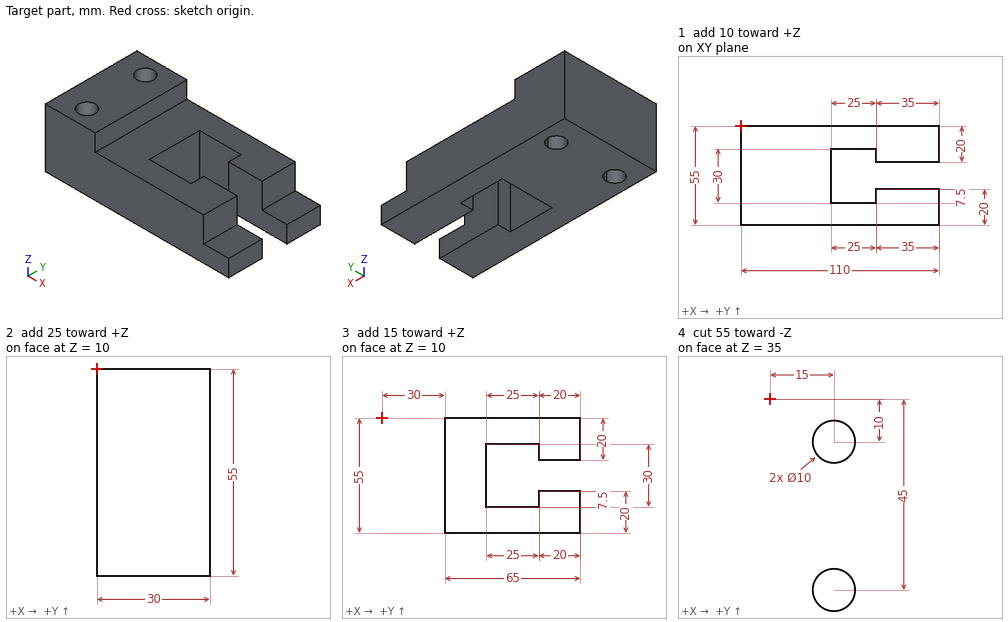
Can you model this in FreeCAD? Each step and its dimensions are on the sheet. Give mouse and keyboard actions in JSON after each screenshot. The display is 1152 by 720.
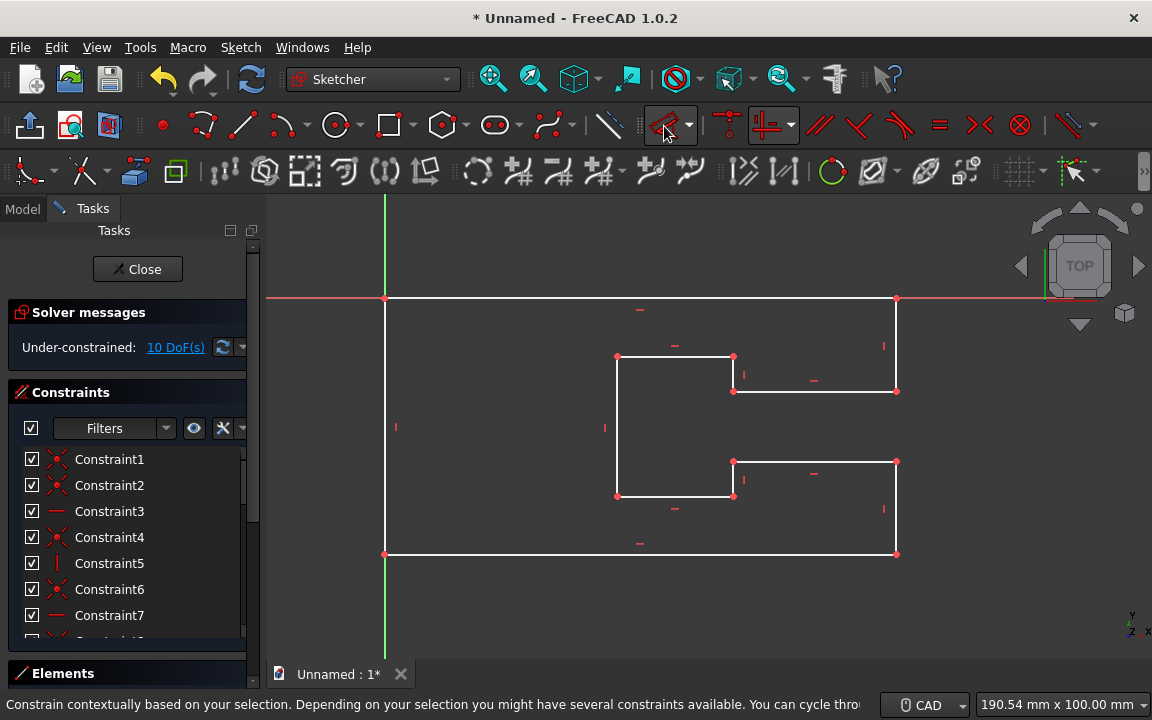
{"action": "left_click", "coordinate": [385, 375]}
{"action": "left_click", "coordinate": [351, 427]}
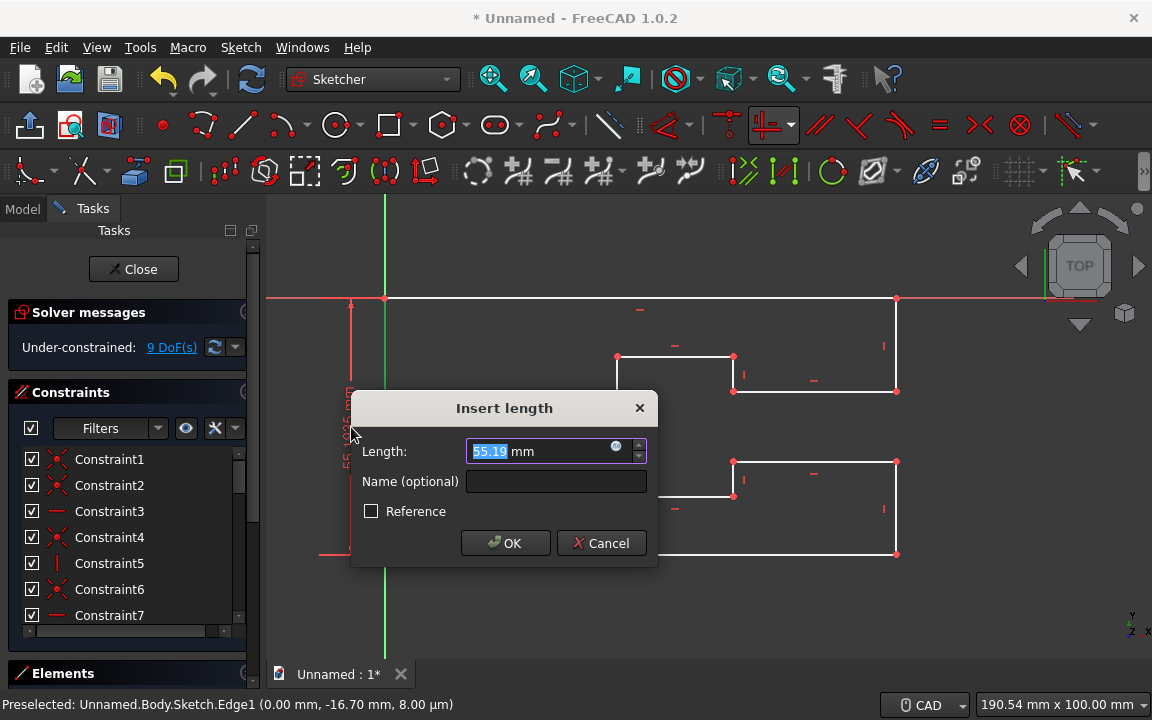
{"action": "type", "text": "55"}
{"action": "key", "text": "Return"}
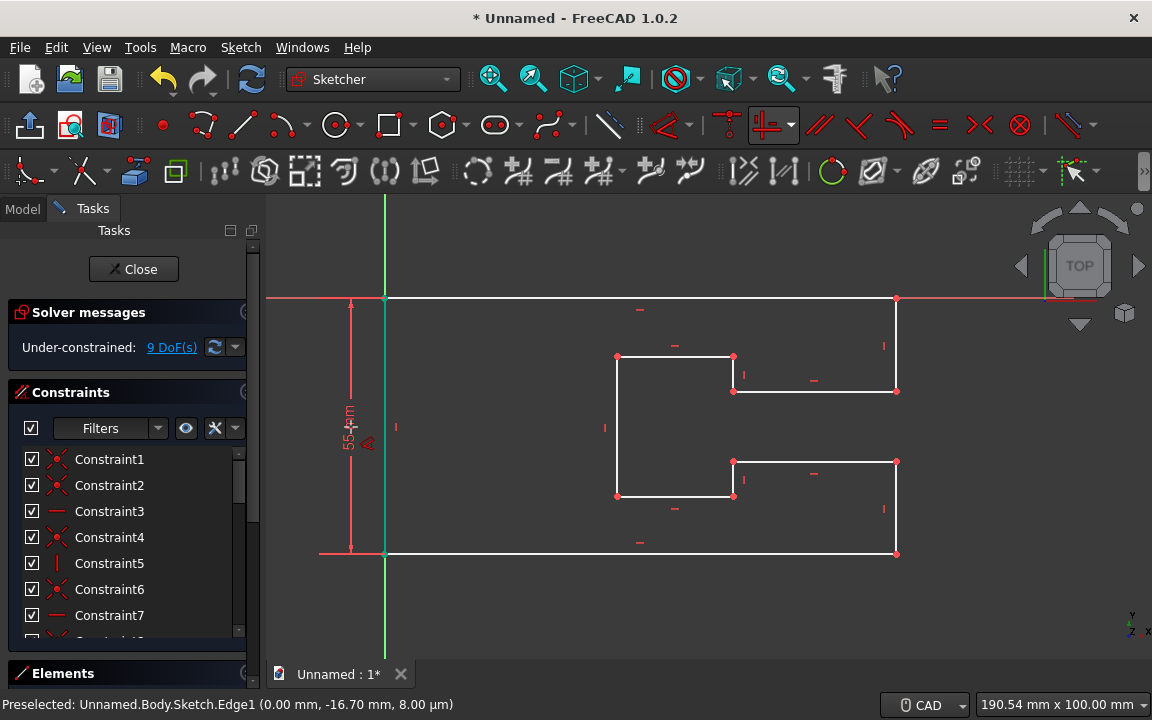
{"action": "left_click", "coordinate": [896, 526]}
{"action": "left_click", "coordinate": [930, 508]}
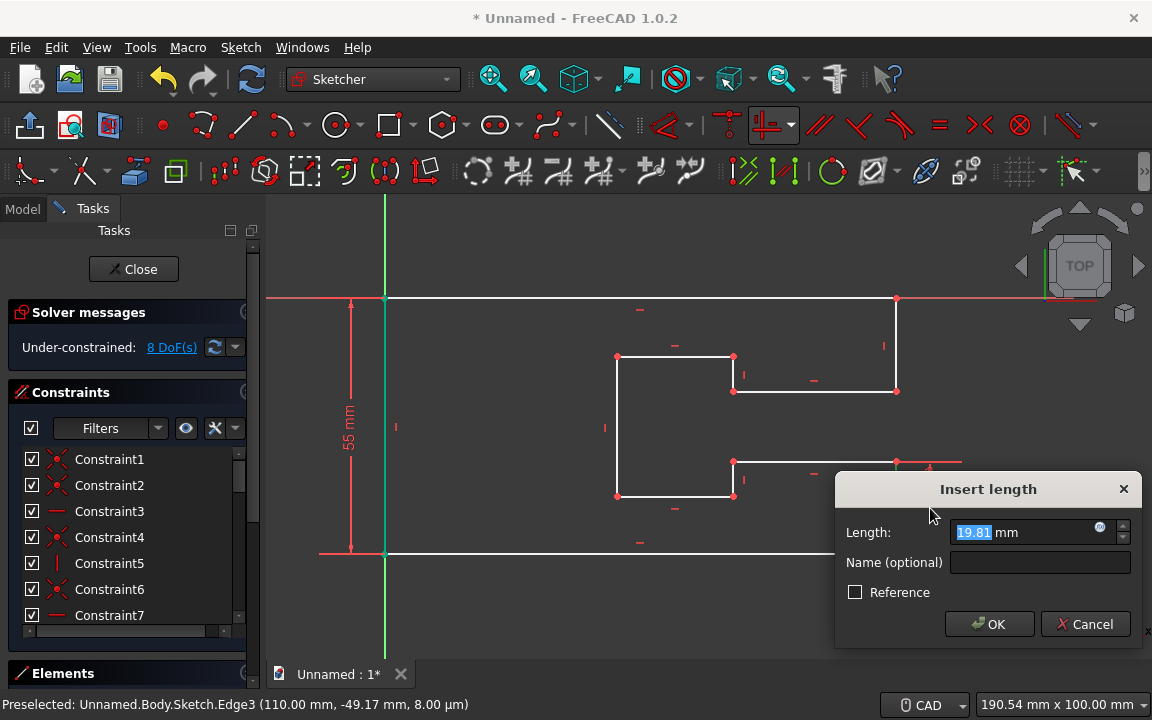
{"action": "type", "text": "20"}
{"action": "key", "text": "Return"}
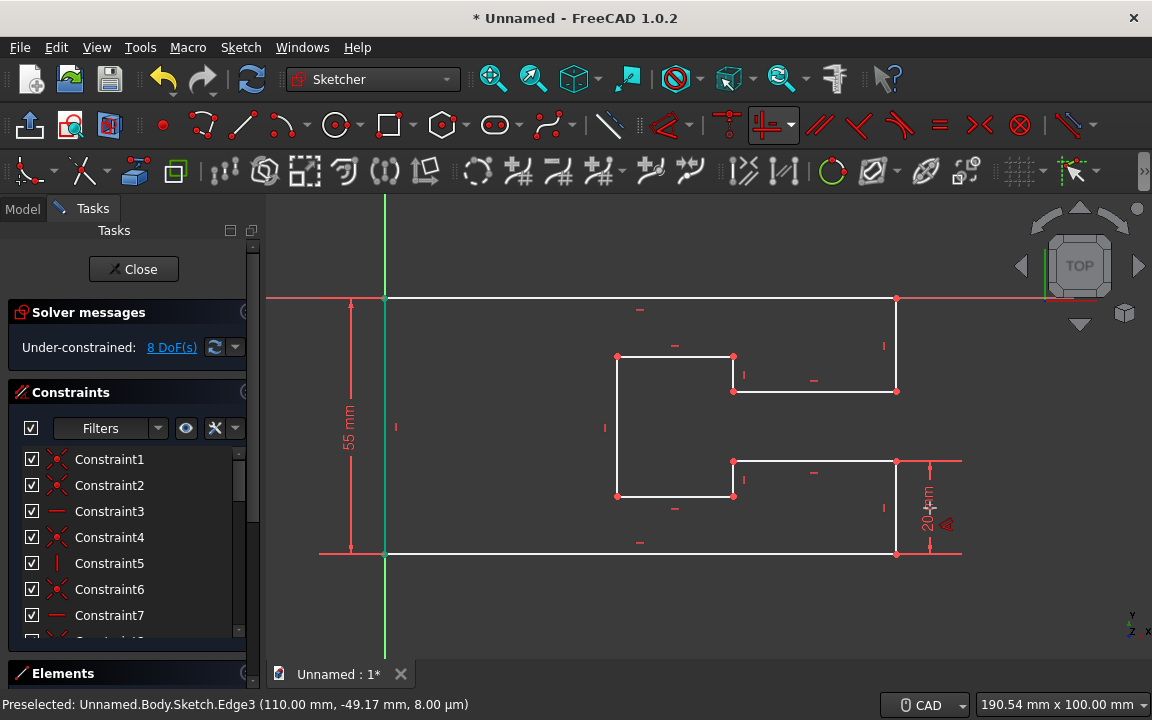
{"action": "left_click", "coordinate": [847, 461]}
{"action": "left_click", "coordinate": [814, 495]}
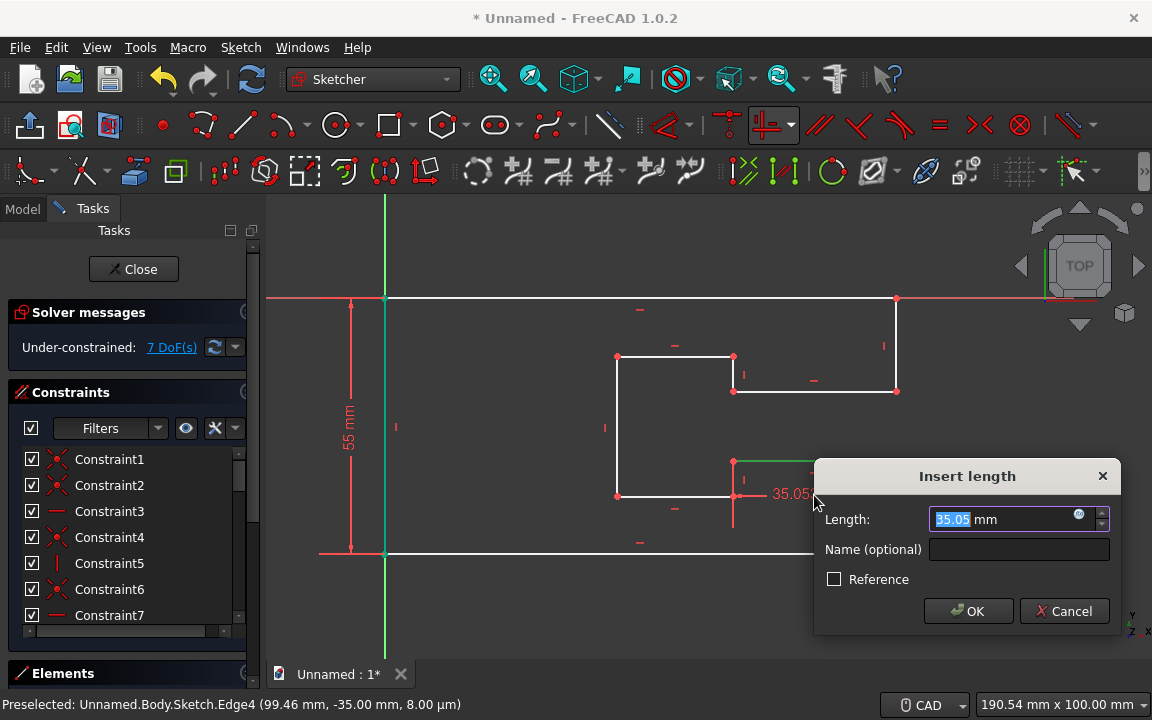
{"action": "type", "text": "35"}
{"action": "key", "text": "Return"}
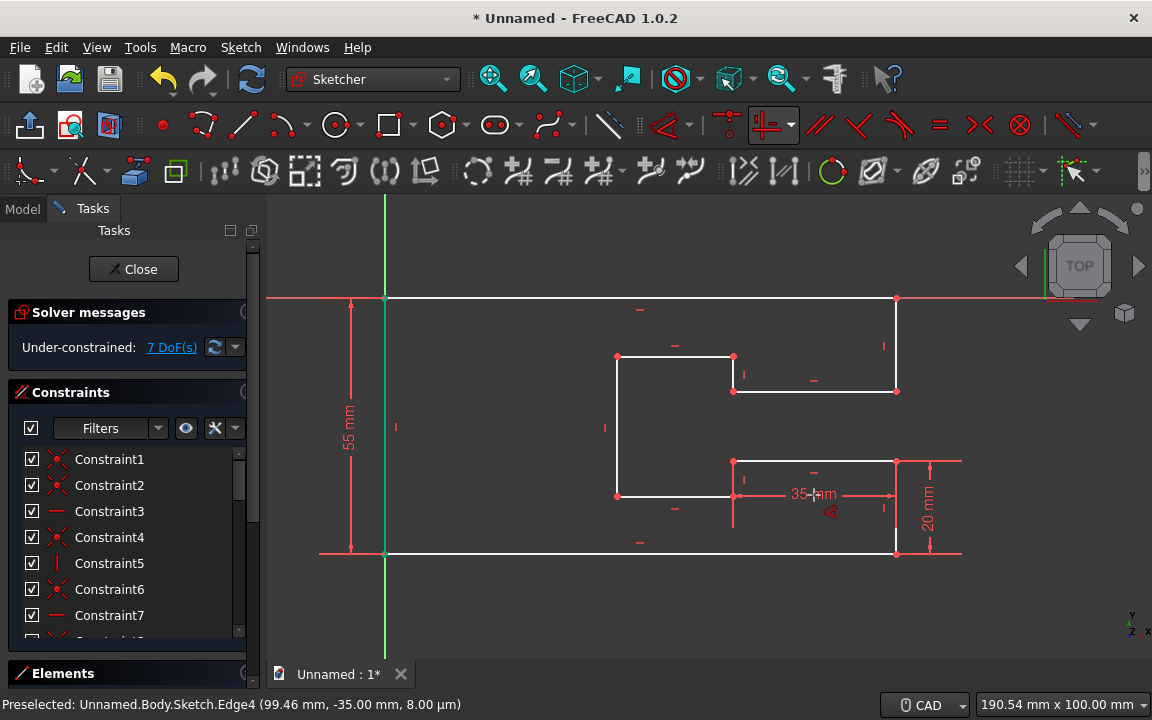
{"action": "left_click", "coordinate": [698, 497]}
{"action": "left_click", "coordinate": [675, 531]}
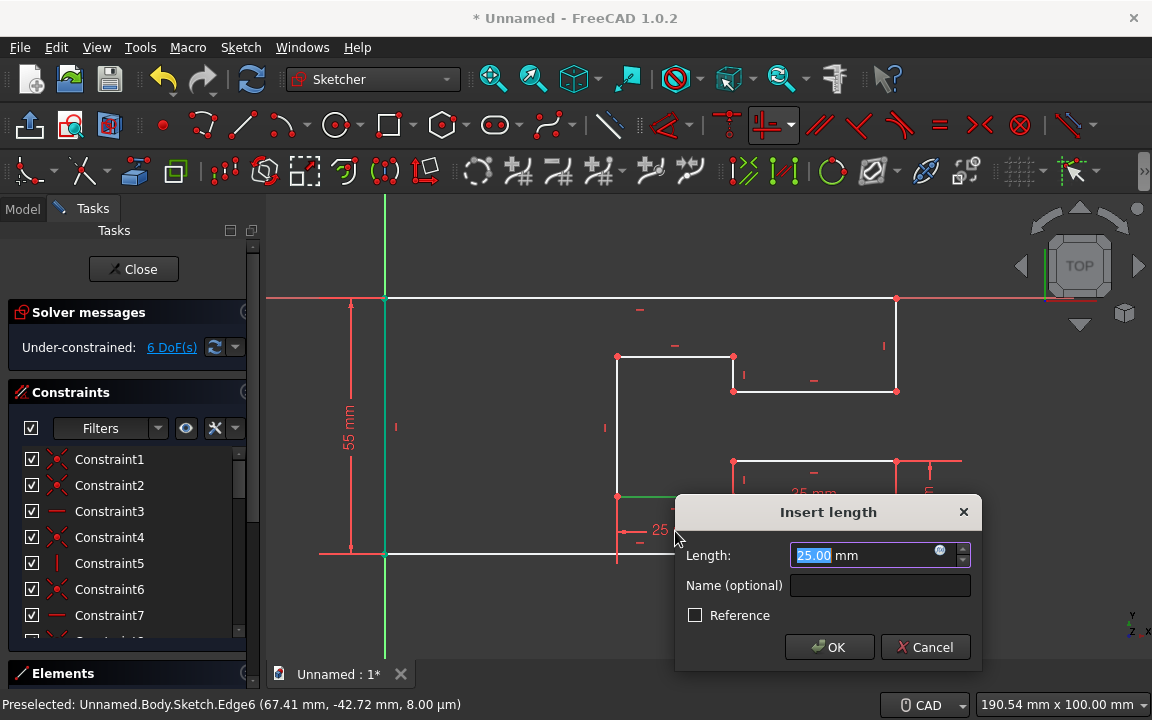
{"action": "type", "text": "25"}
{"action": "key", "text": "Return"}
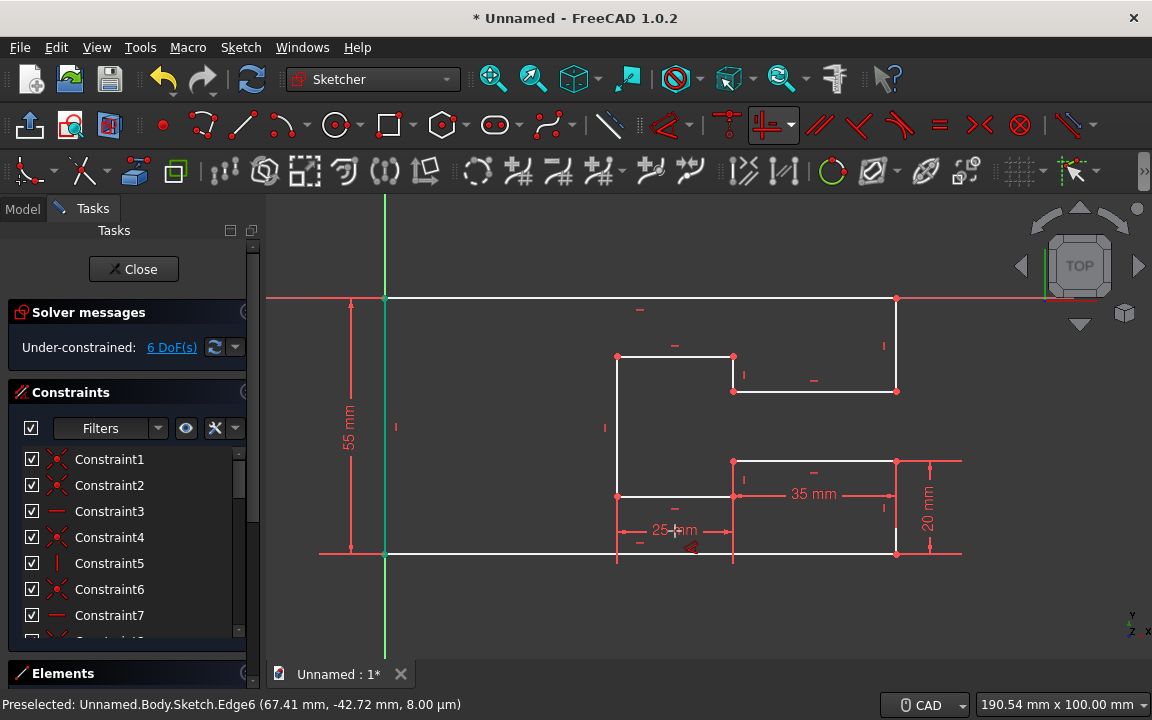
{"action": "left_click", "coordinate": [617, 455]}
{"action": "left_click", "coordinate": [583, 427]}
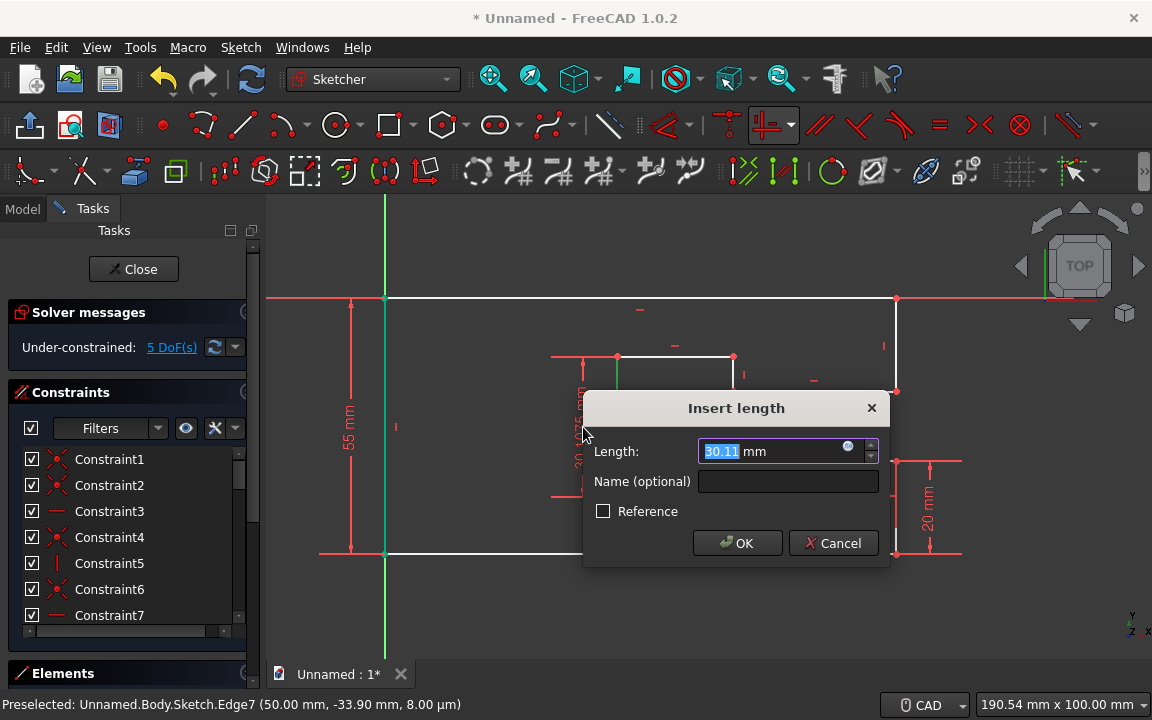
{"action": "type", "text": "30"}
{"action": "key", "text": "Return"}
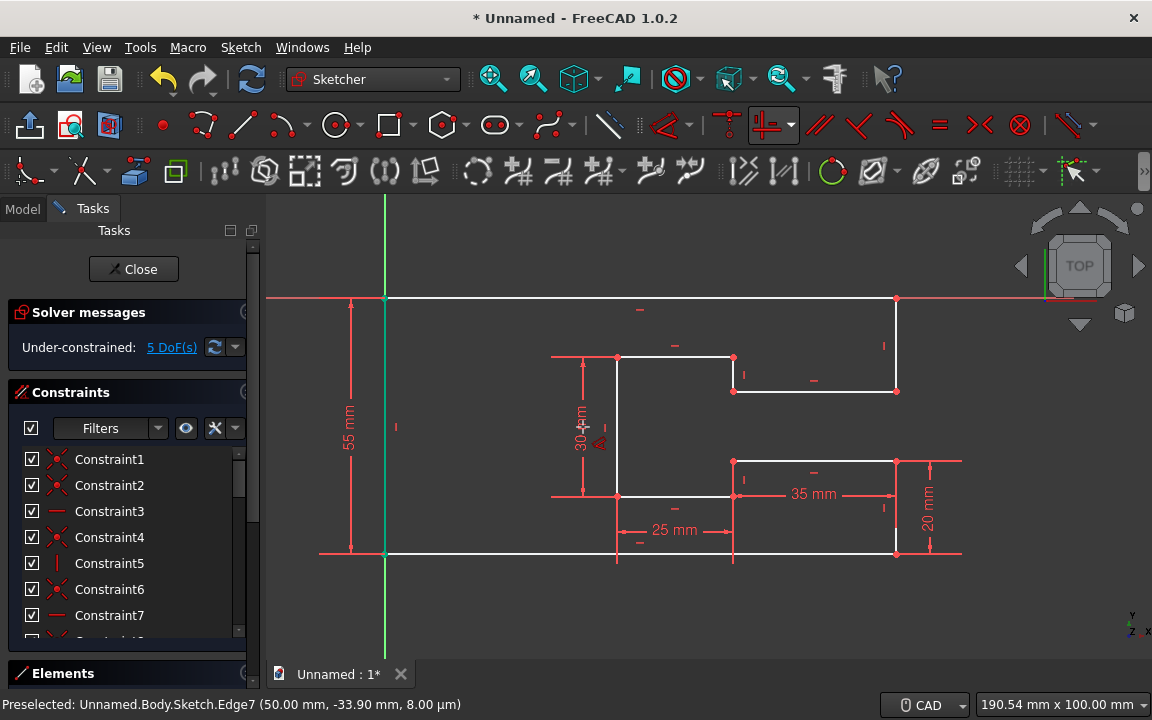
{"action": "left_click", "coordinate": [652, 357]}
{"action": "left_click", "coordinate": [675, 323]}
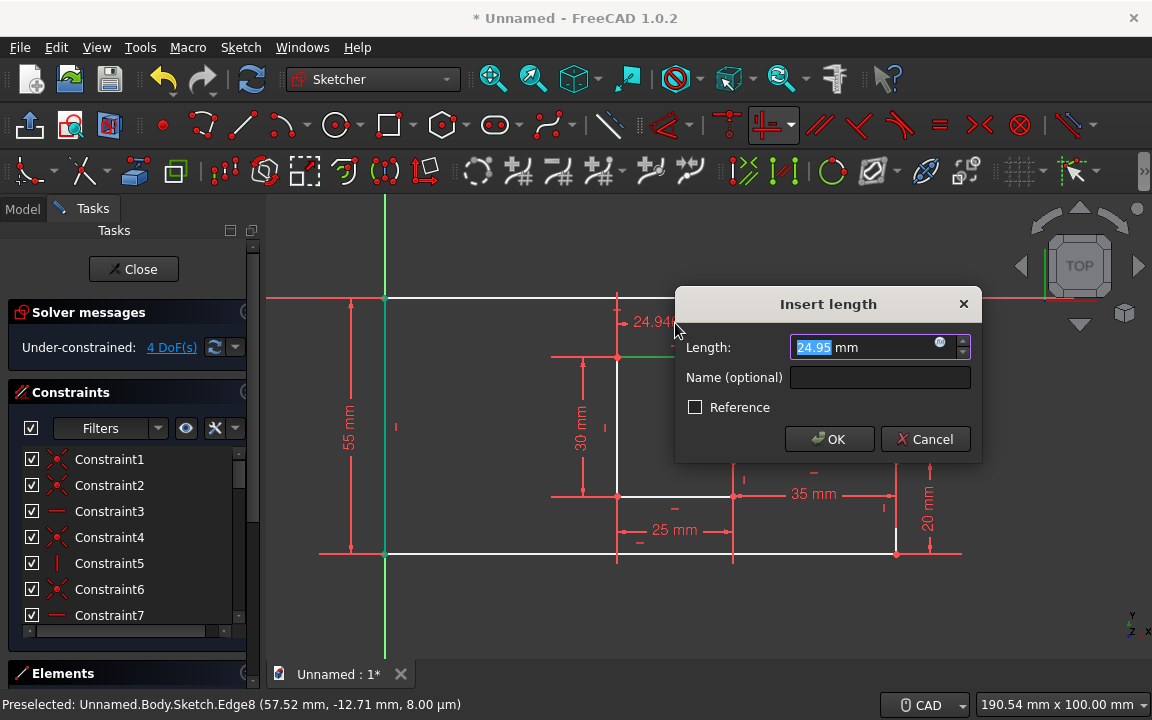
{"action": "type", "text": "25"}
{"action": "key", "text": "Return"}